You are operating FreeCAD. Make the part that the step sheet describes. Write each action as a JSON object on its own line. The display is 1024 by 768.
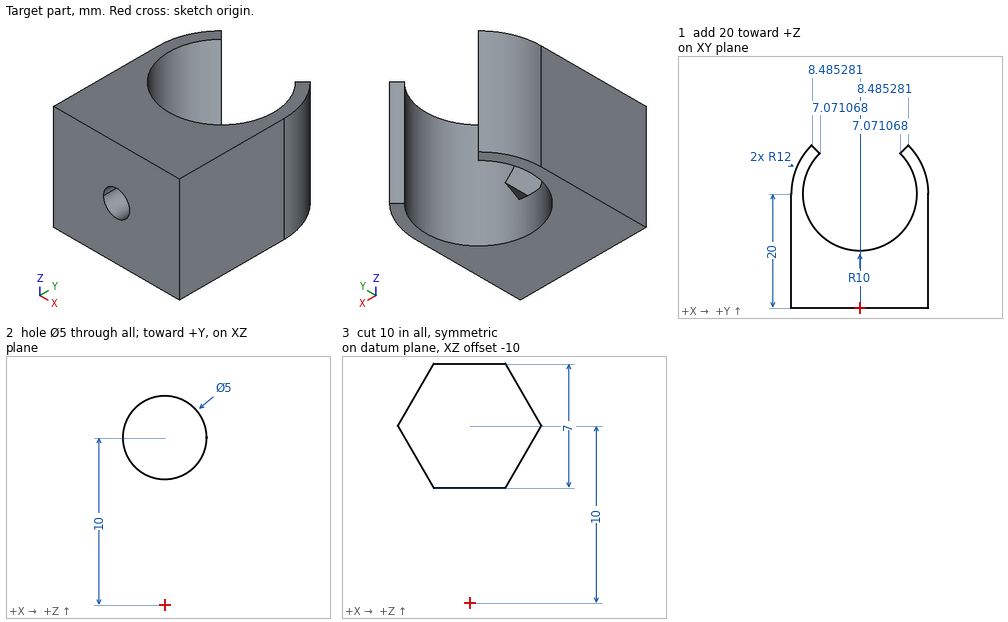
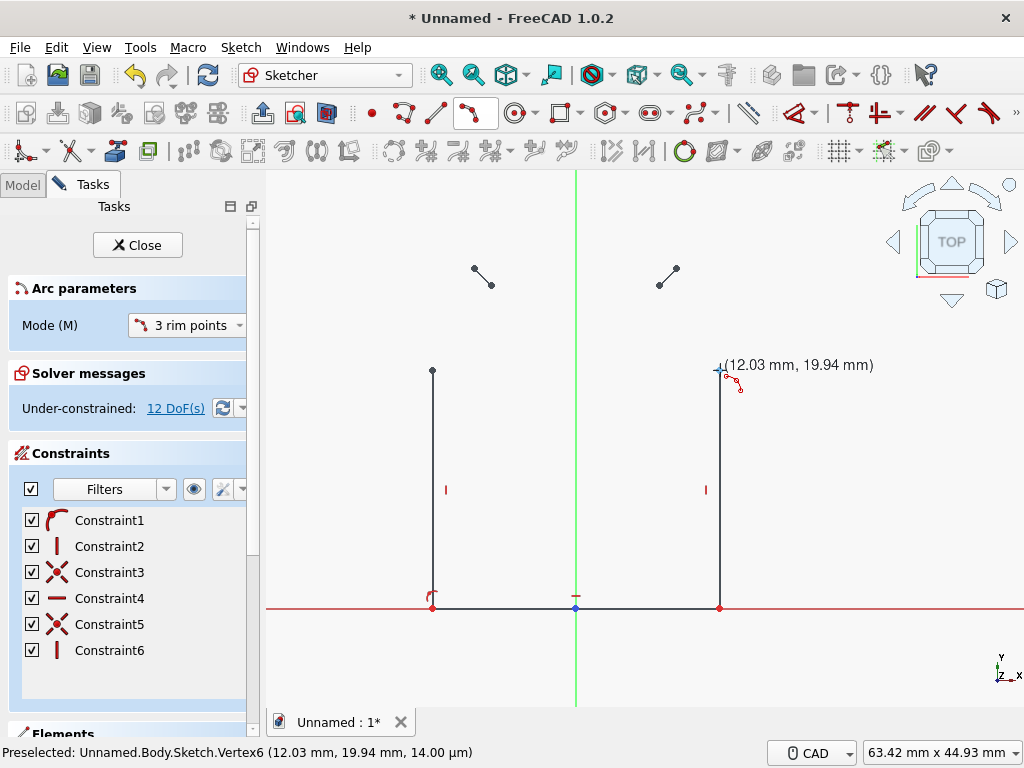
{"action": "scroll", "coordinate": [677, 268], "scroll_direction": "up", "scroll_amount": 2}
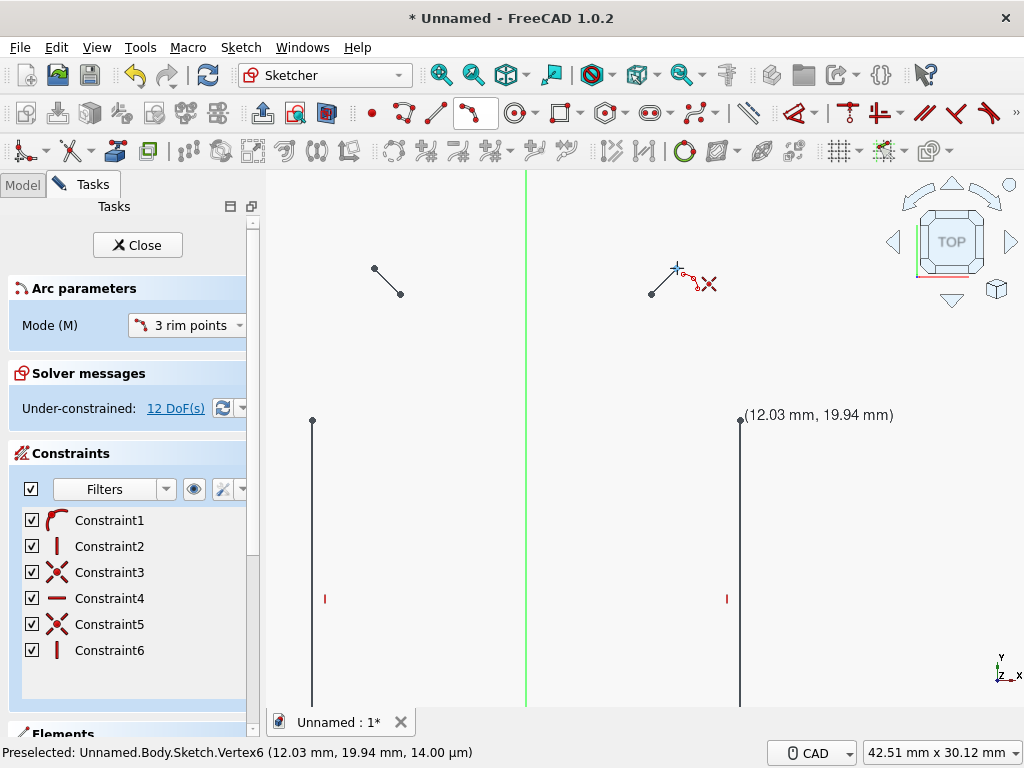
{"action": "left_click", "coordinate": [677, 269]}
{"action": "left_click", "coordinate": [724, 337]}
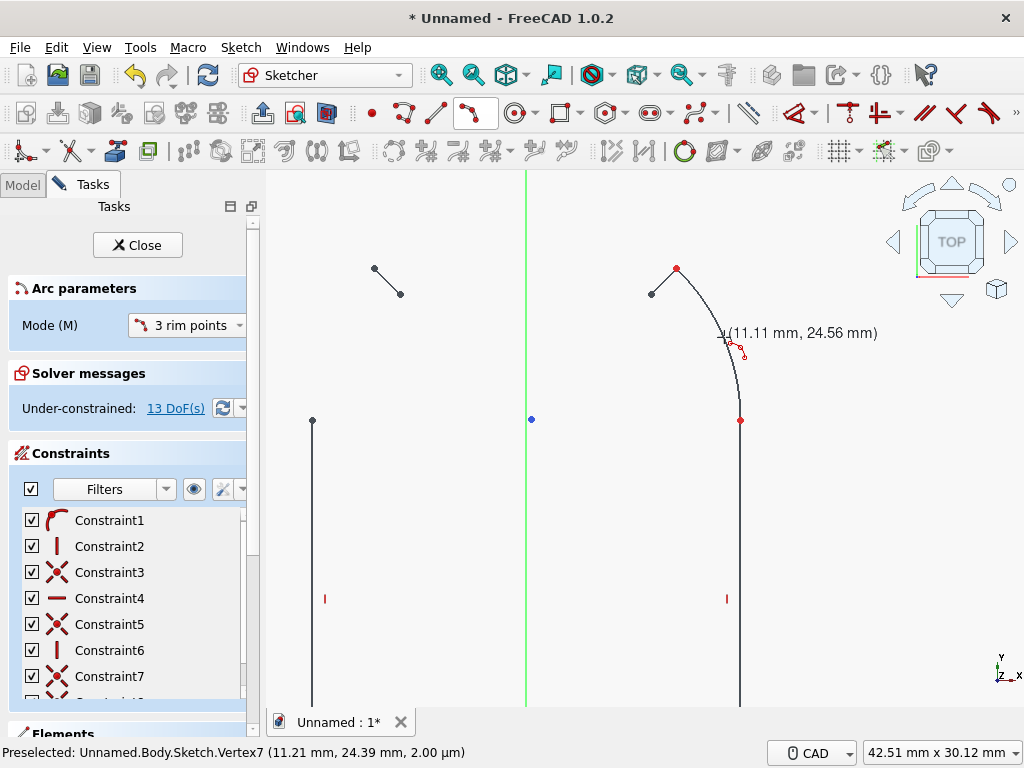
{"action": "left_click", "coordinate": [651, 294]}
{"action": "left_click", "coordinate": [400, 294]}
{"action": "left_click", "coordinate": [445, 578]}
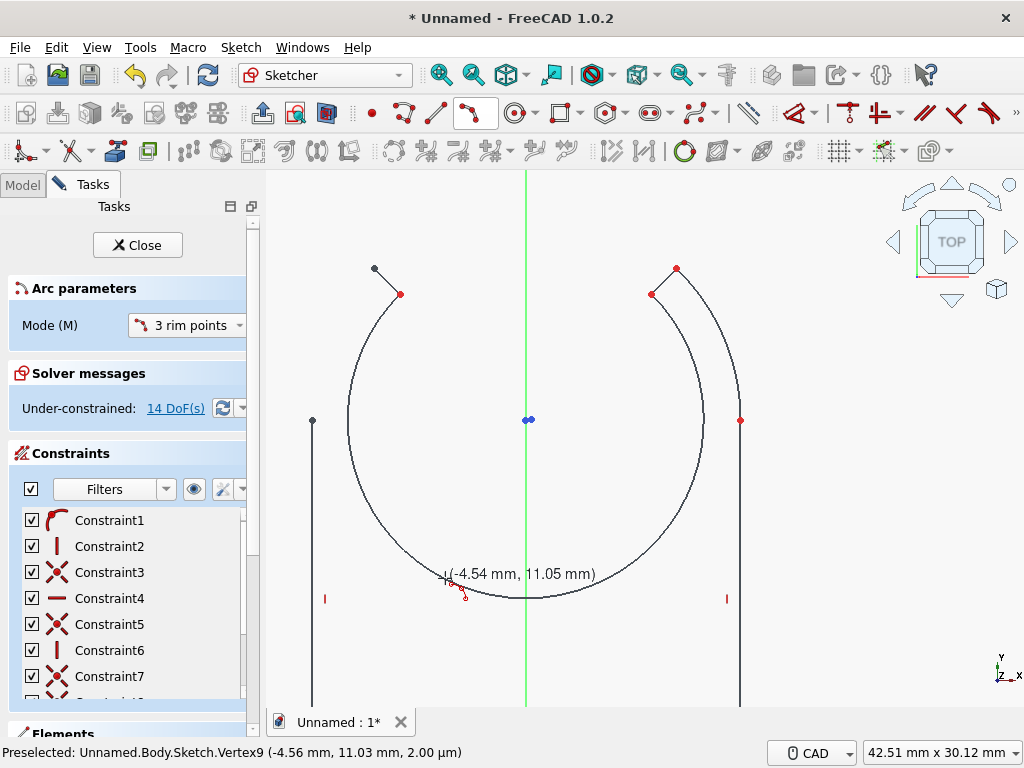
{"action": "left_click", "coordinate": [375, 269]}
{"action": "left_click", "coordinate": [312, 420]}
{"action": "left_click", "coordinate": [328, 337]}
{"action": "key", "text": "Escape"}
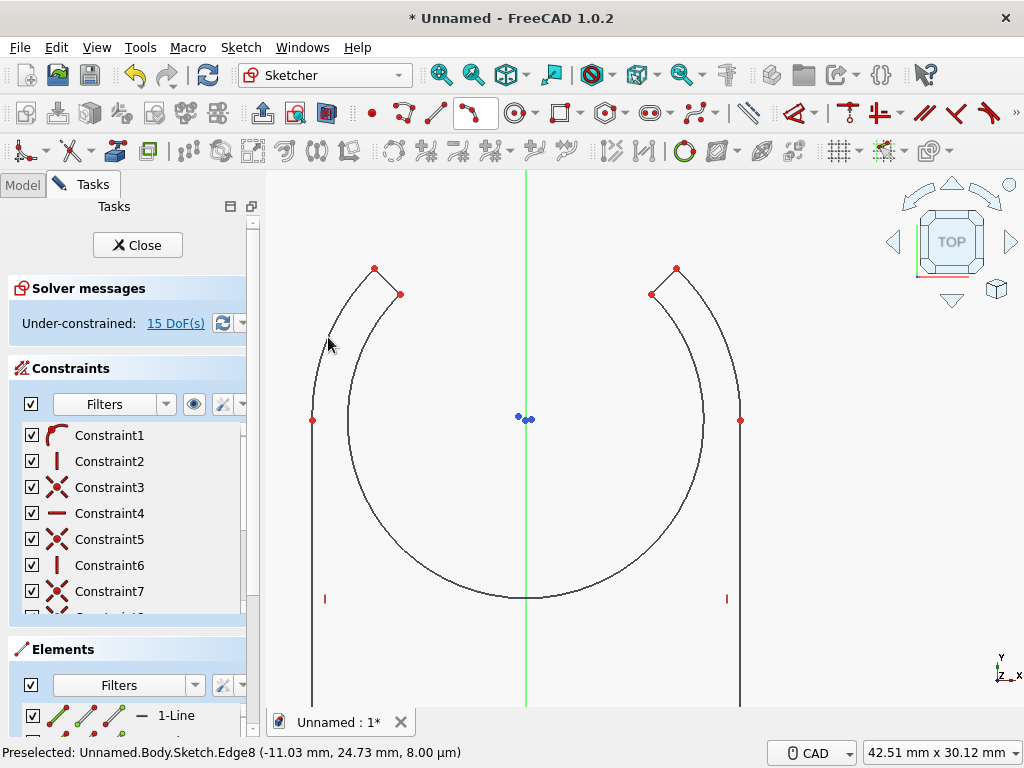
{"action": "left_click", "coordinate": [312, 527]}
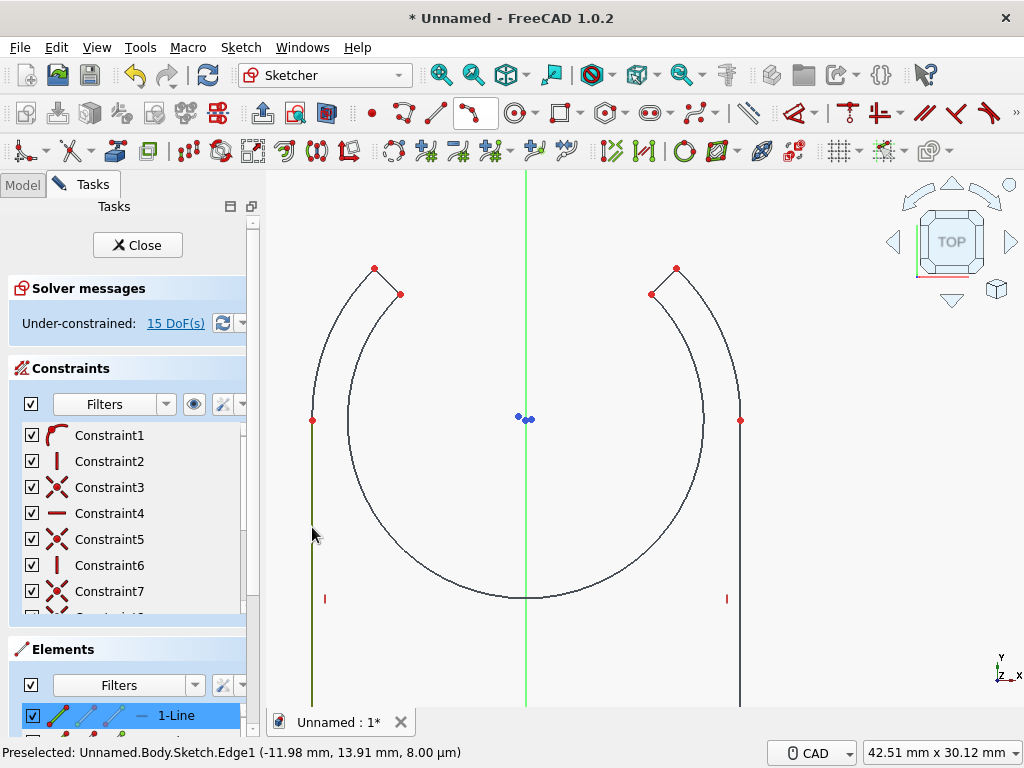
{"action": "left_click", "coordinate": [343, 308]}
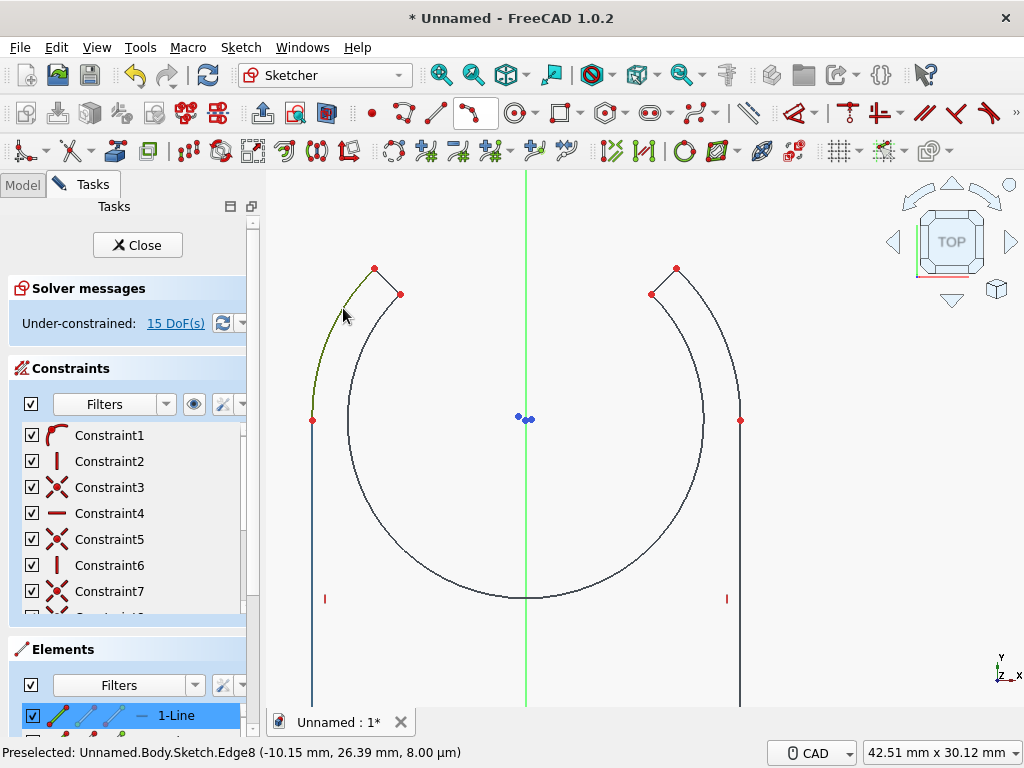
{"action": "left_click", "coordinate": [990, 114]}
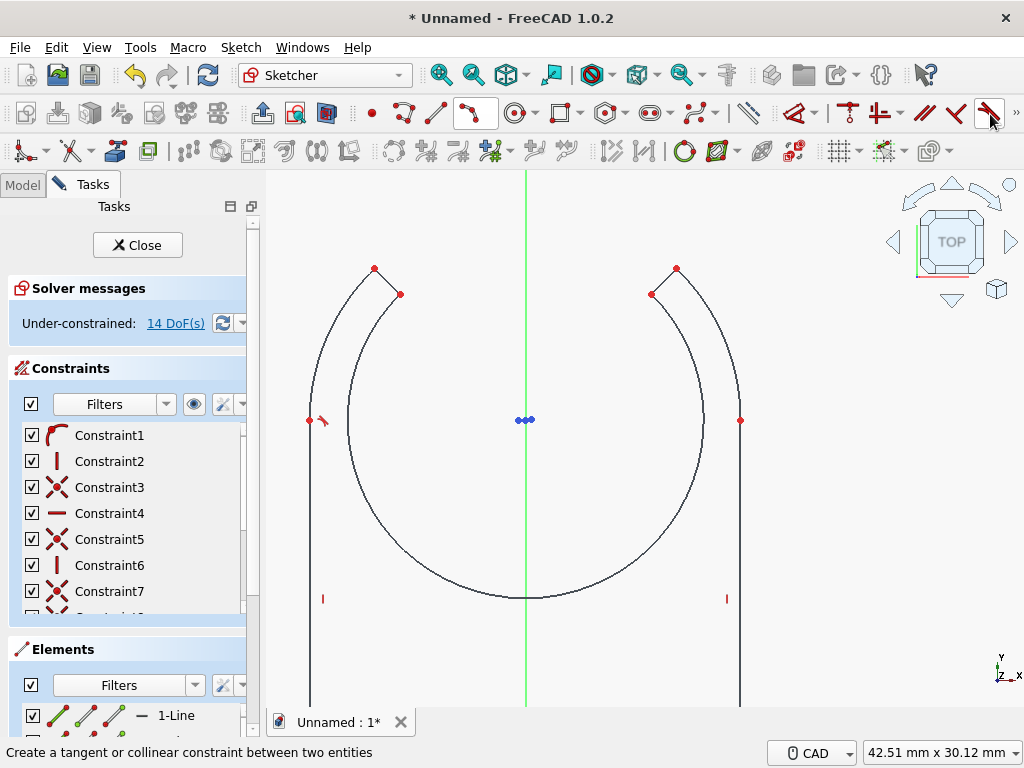
{"action": "left_click", "coordinate": [740, 669]}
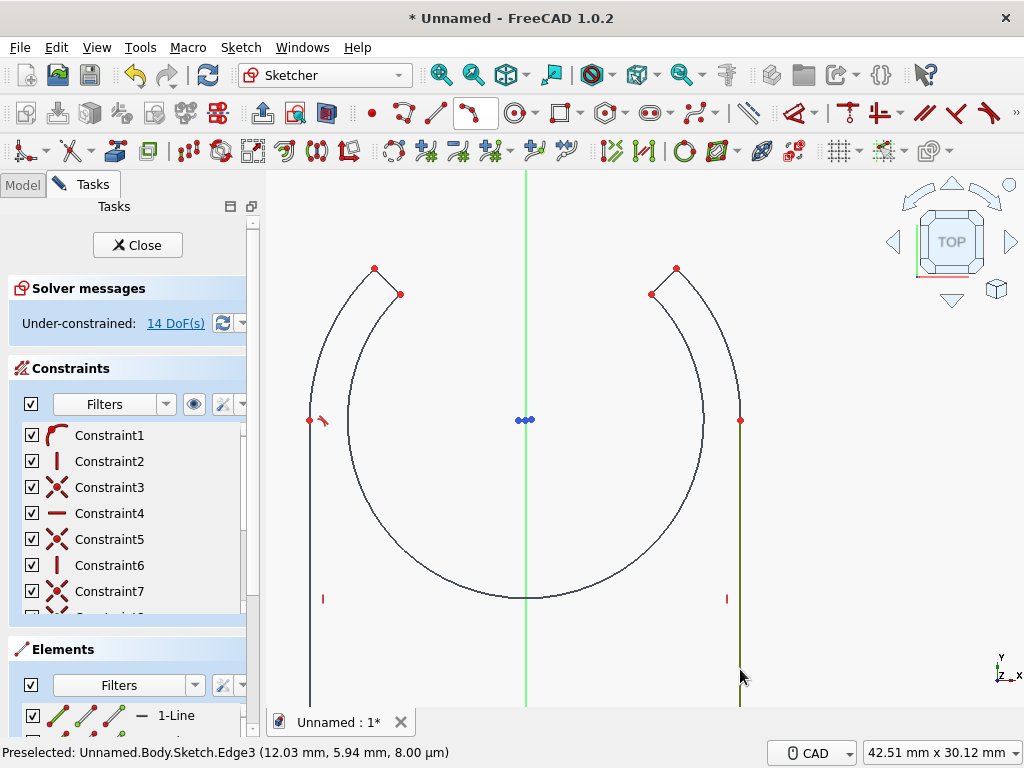
{"action": "left_click", "coordinate": [735, 370]}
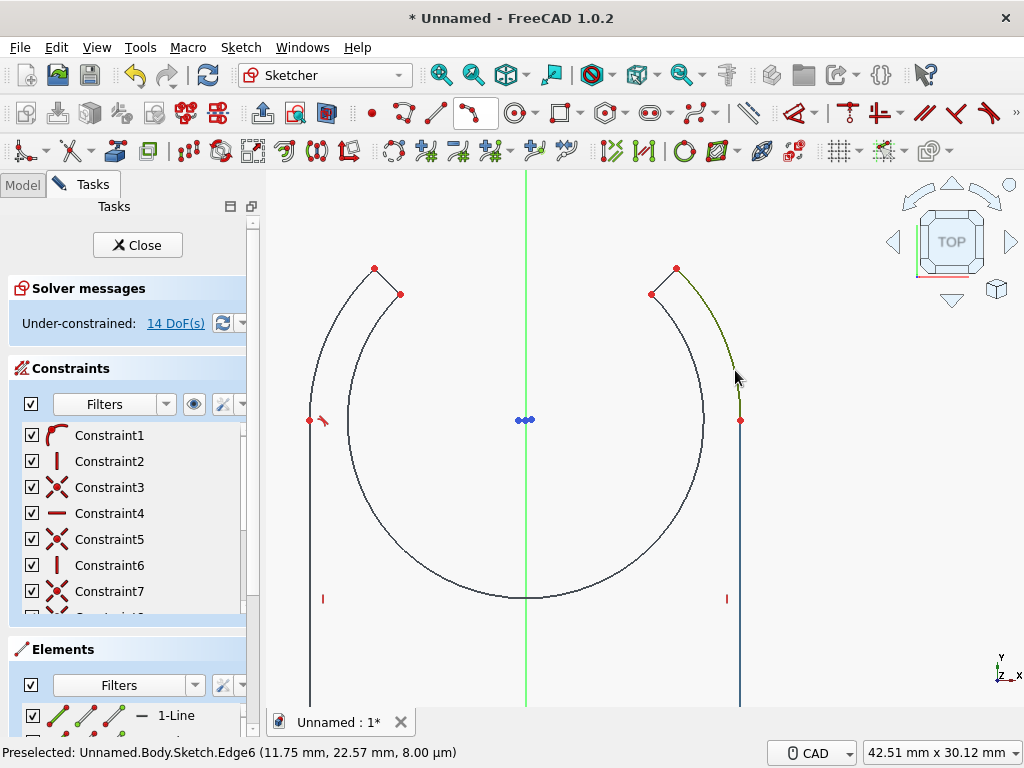
{"action": "left_click", "coordinate": [990, 114]}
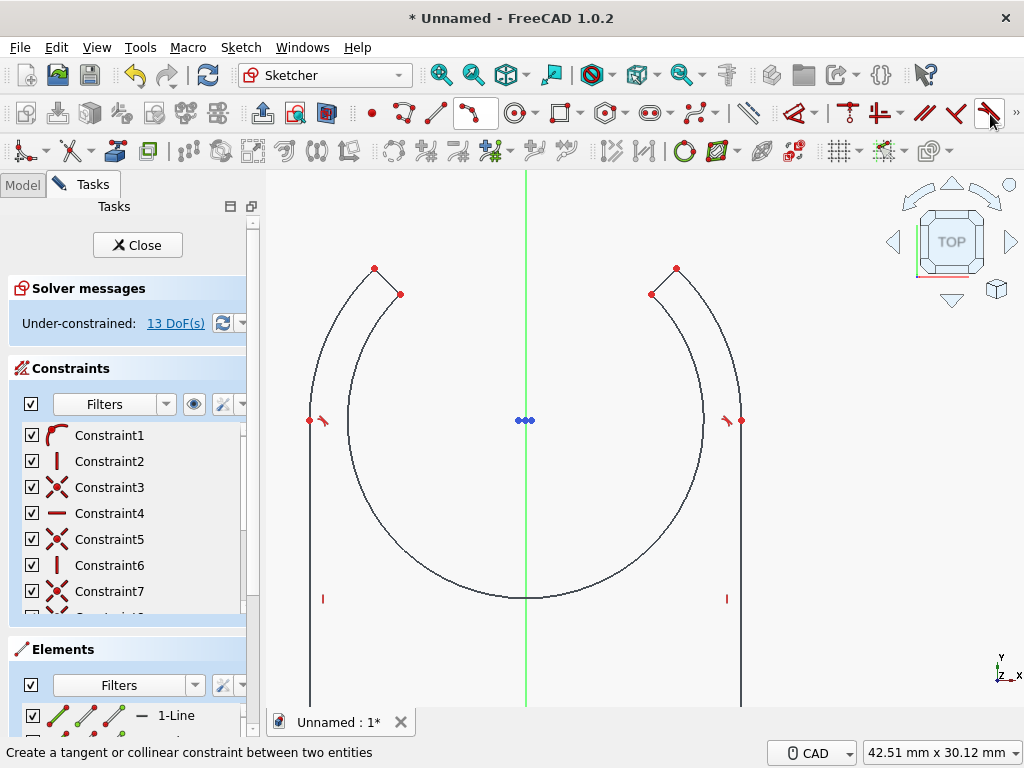
{"action": "left_click", "coordinate": [735, 370]}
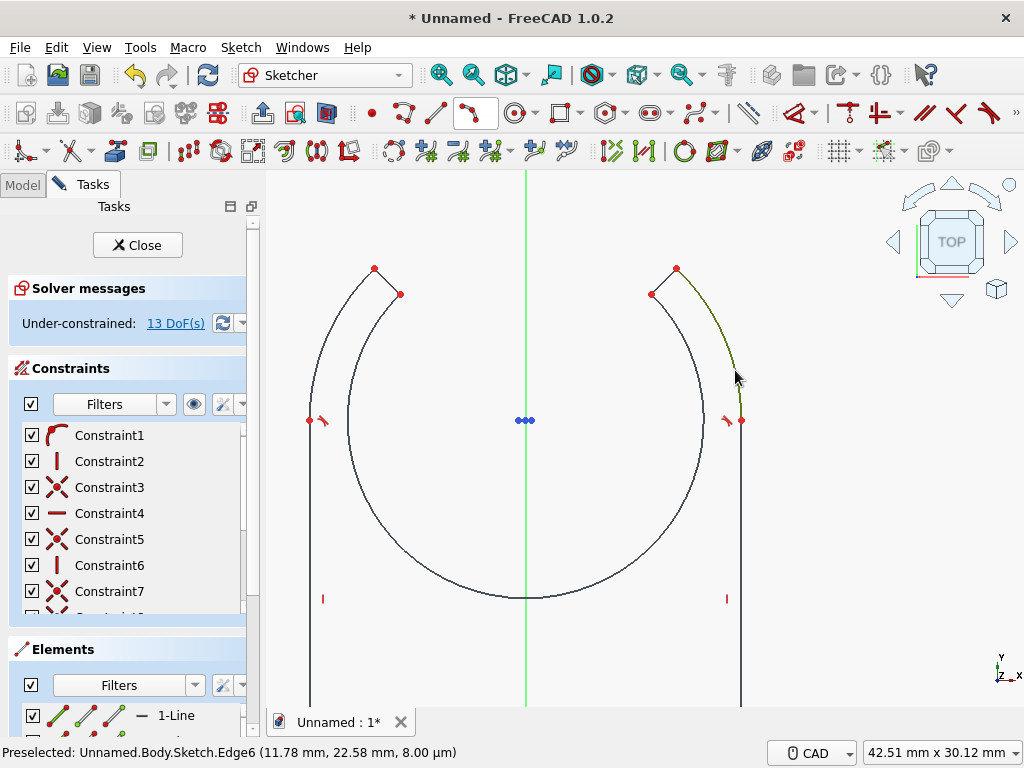
{"action": "left_click", "coordinate": [382, 525]}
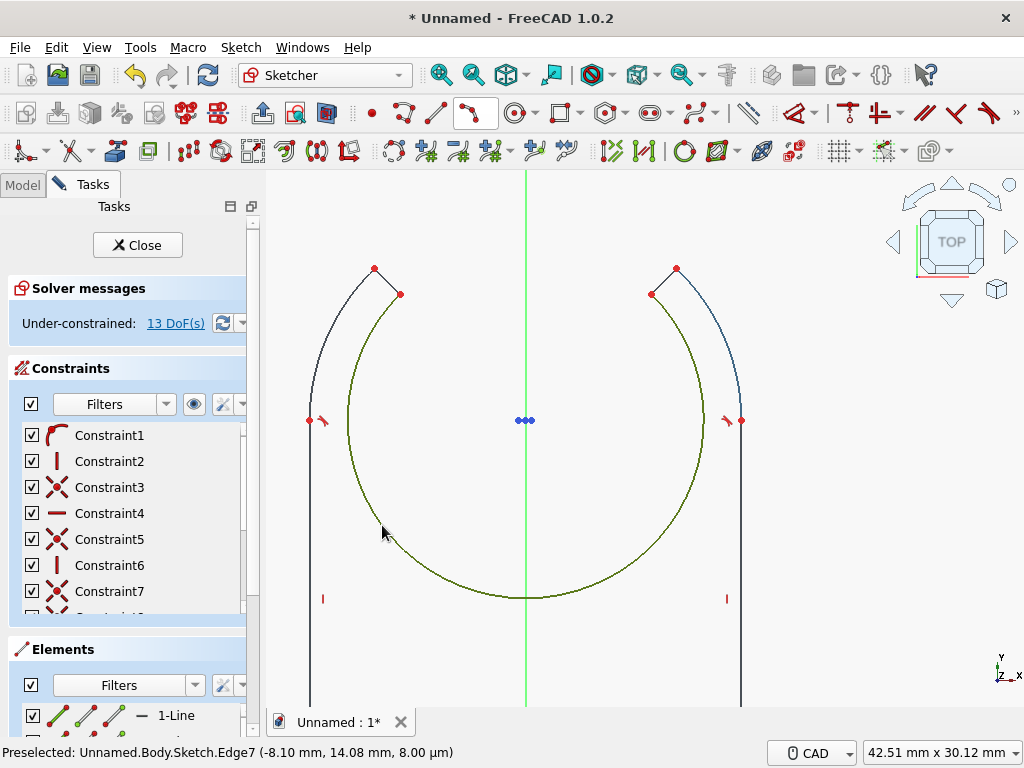
{"action": "left_click", "coordinate": [848, 114]}